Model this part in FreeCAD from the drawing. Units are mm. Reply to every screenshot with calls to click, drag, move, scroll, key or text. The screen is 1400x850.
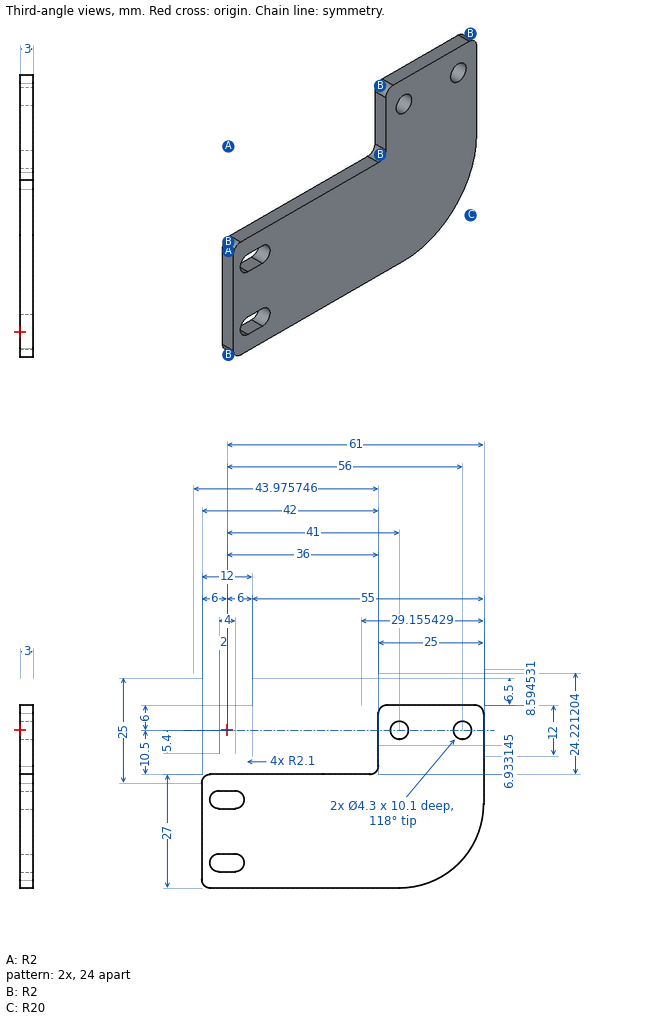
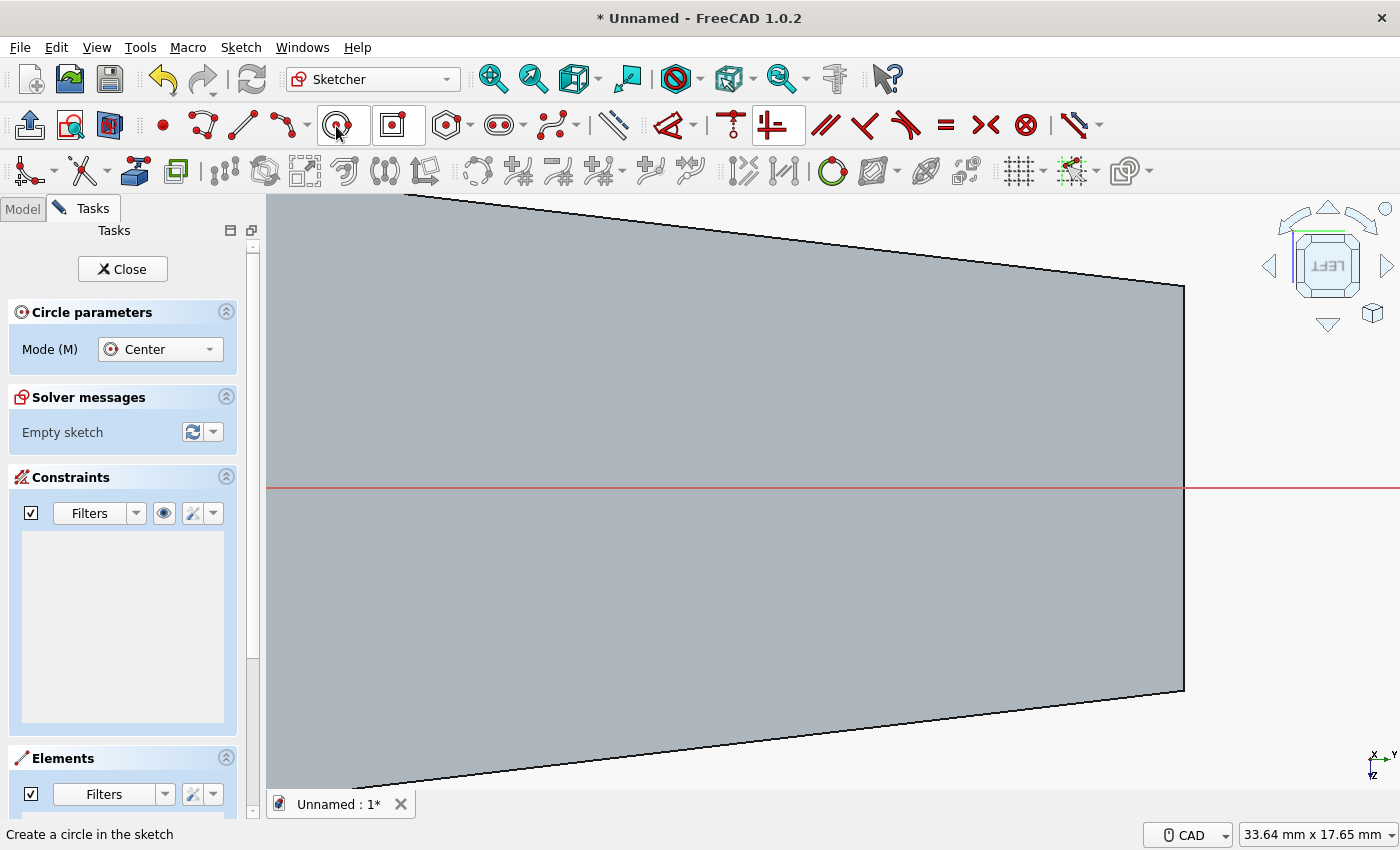
click(1016, 488)
move(1067, 437)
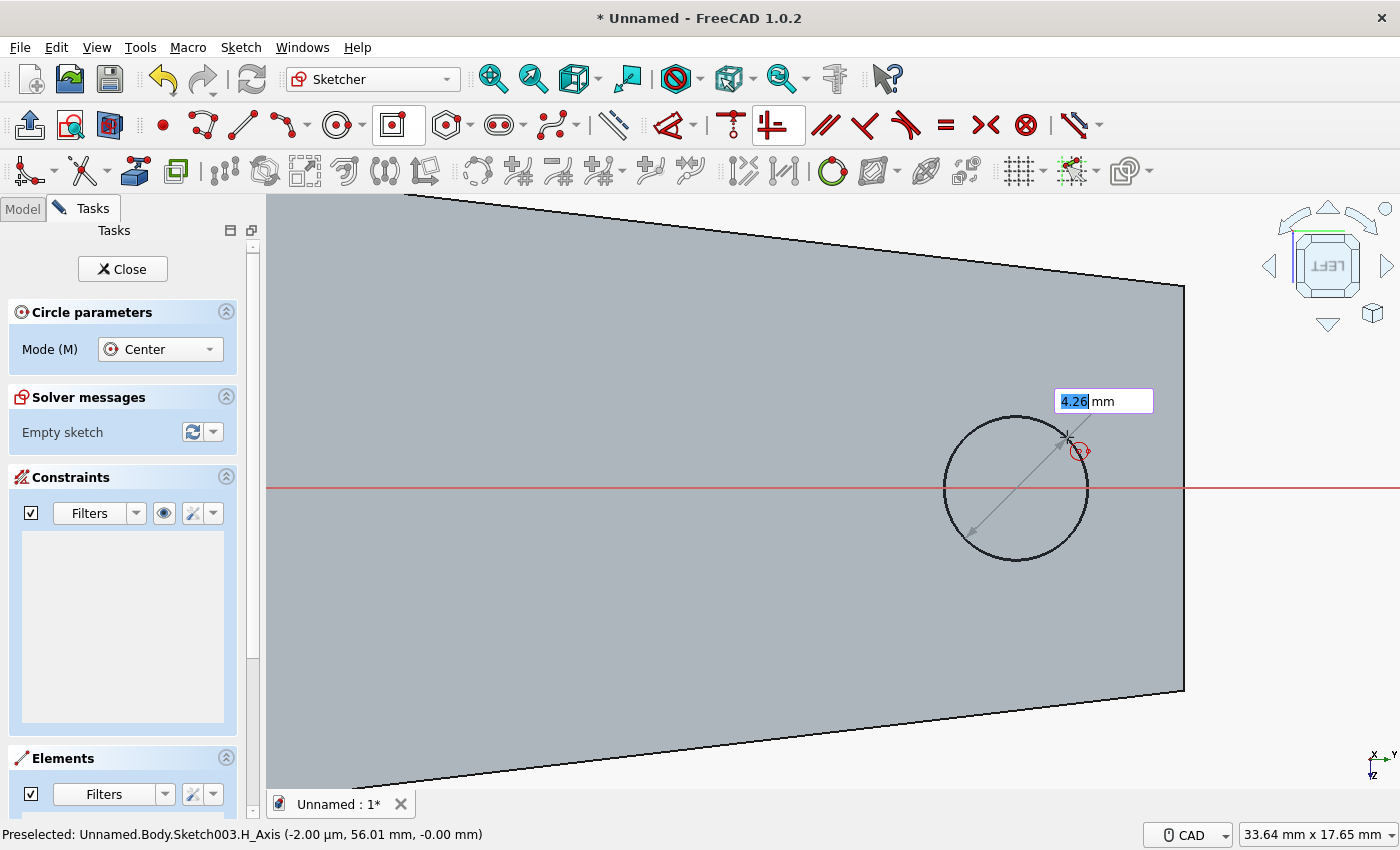
text(4.3)
key(Return)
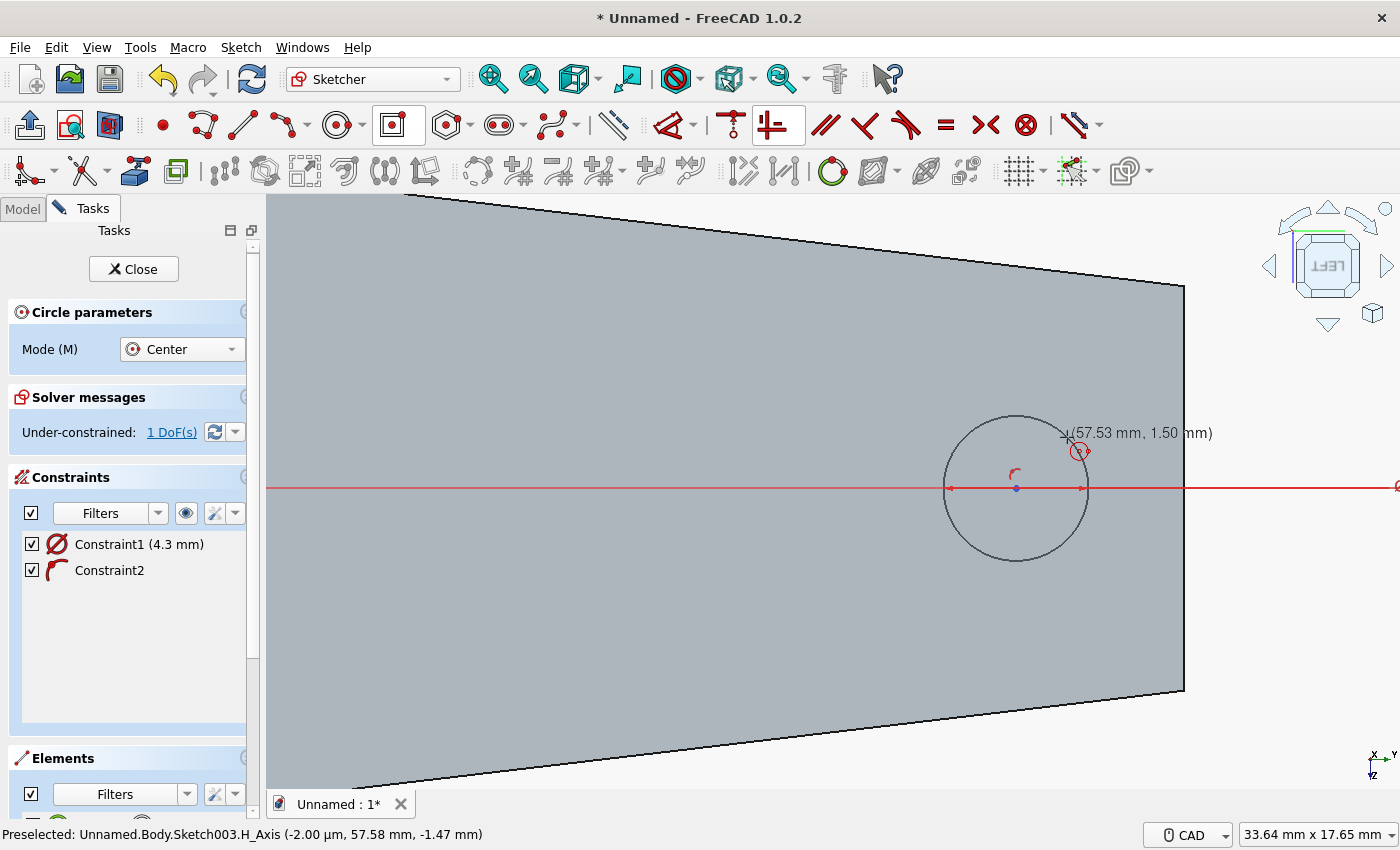
click(510, 488)
move(561, 437)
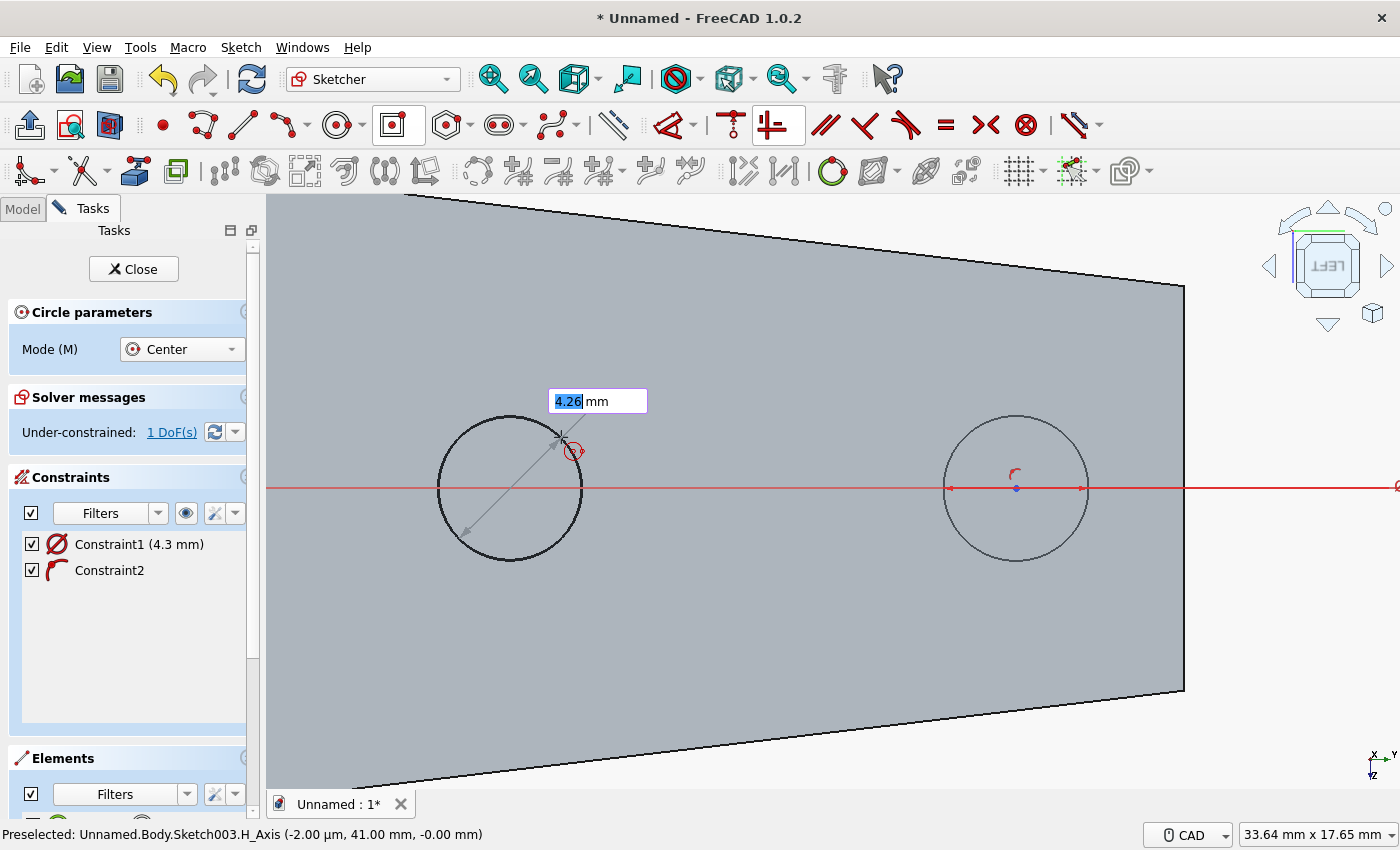
text(4.3)
key(Return)
key(Escape)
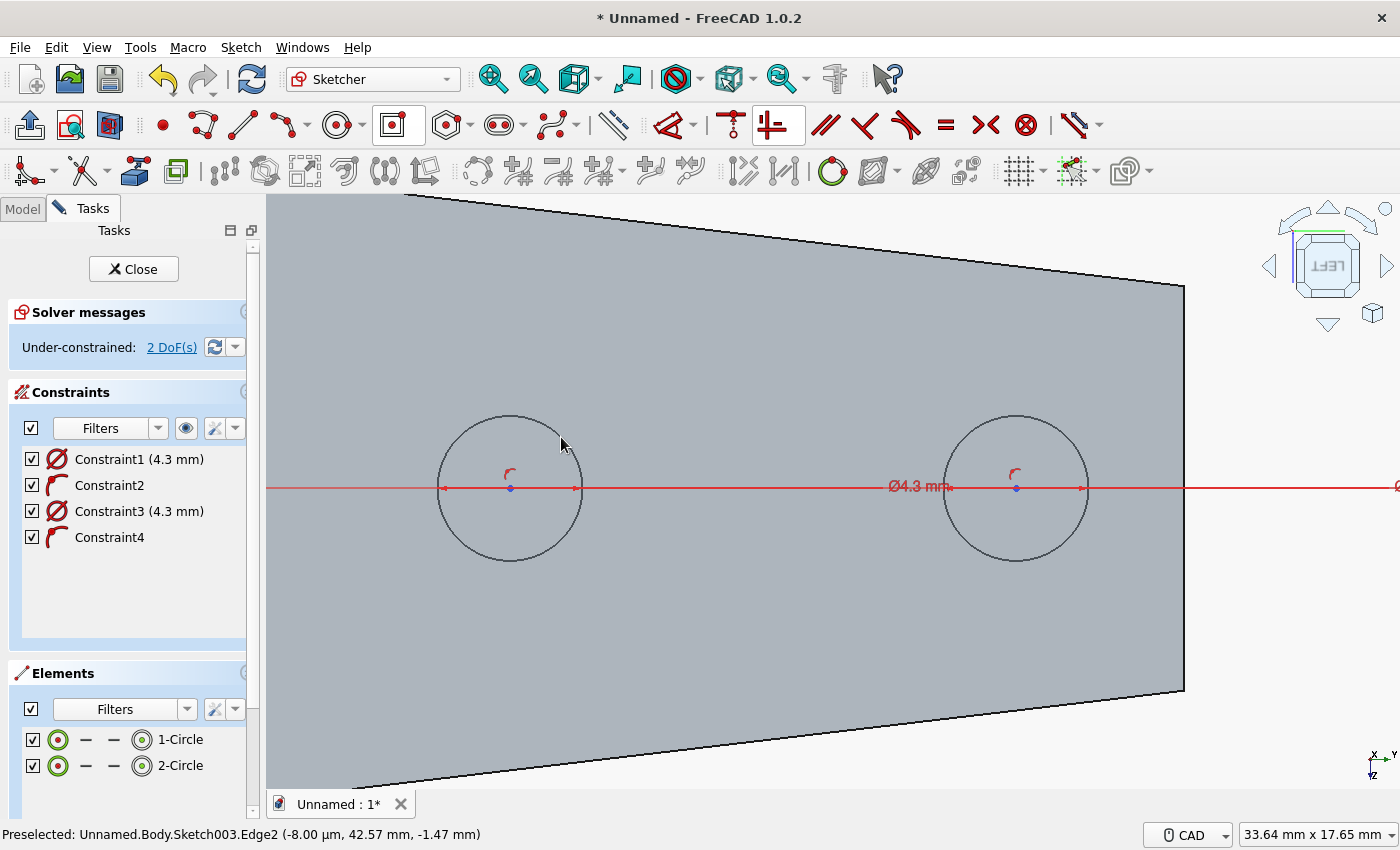
key(d)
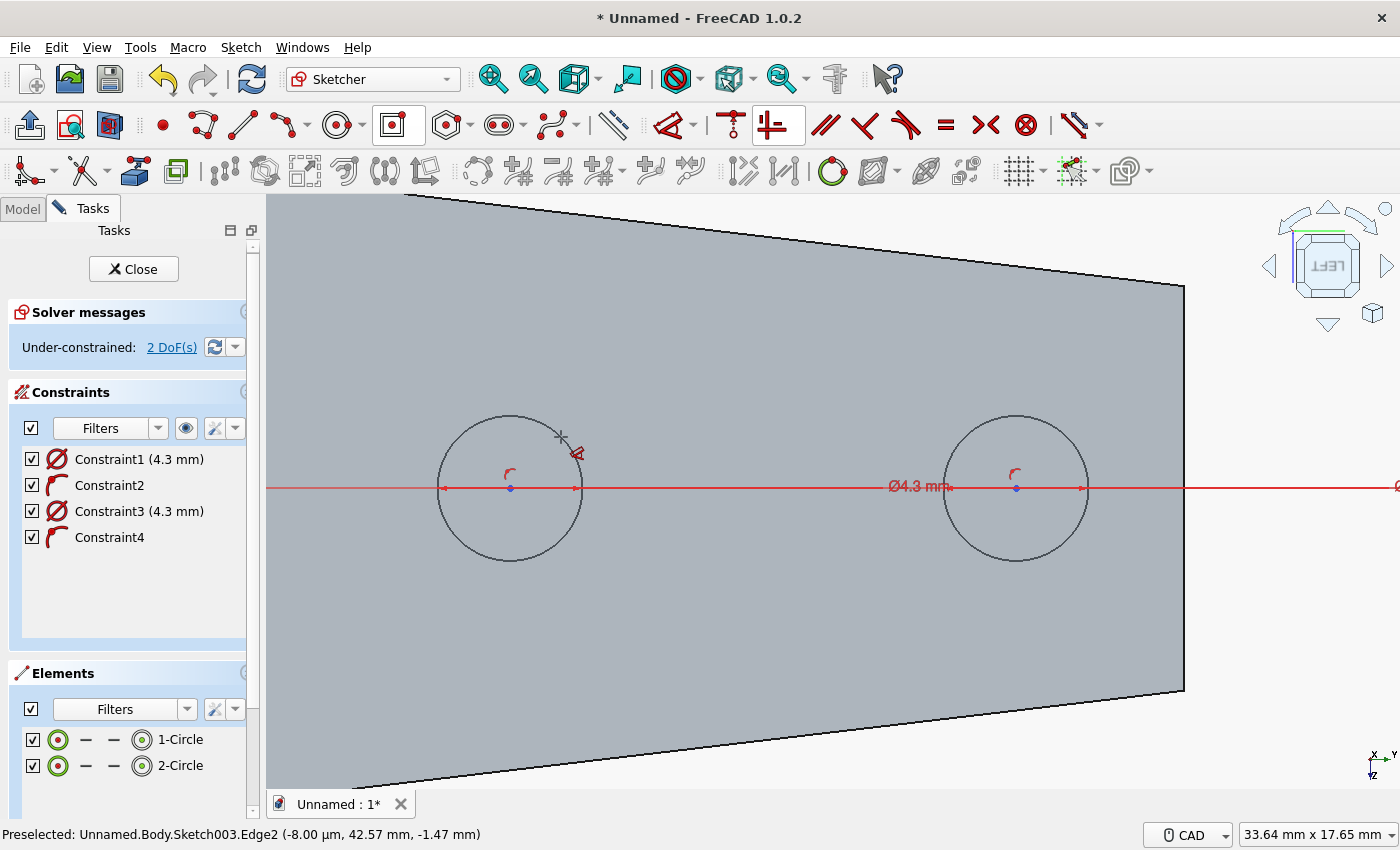
click(1016, 488)
click(655, 522)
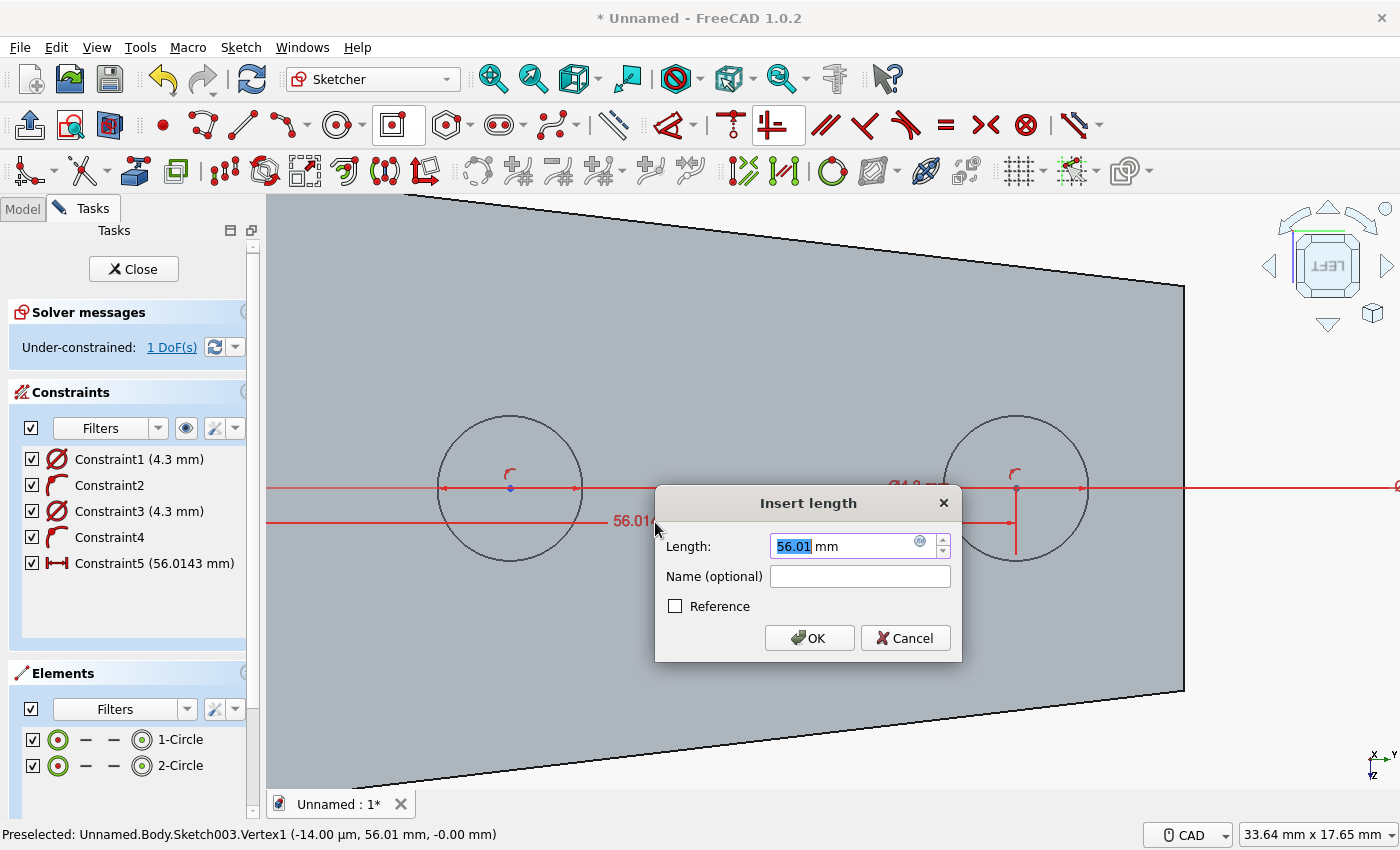
text(56)
key(Return)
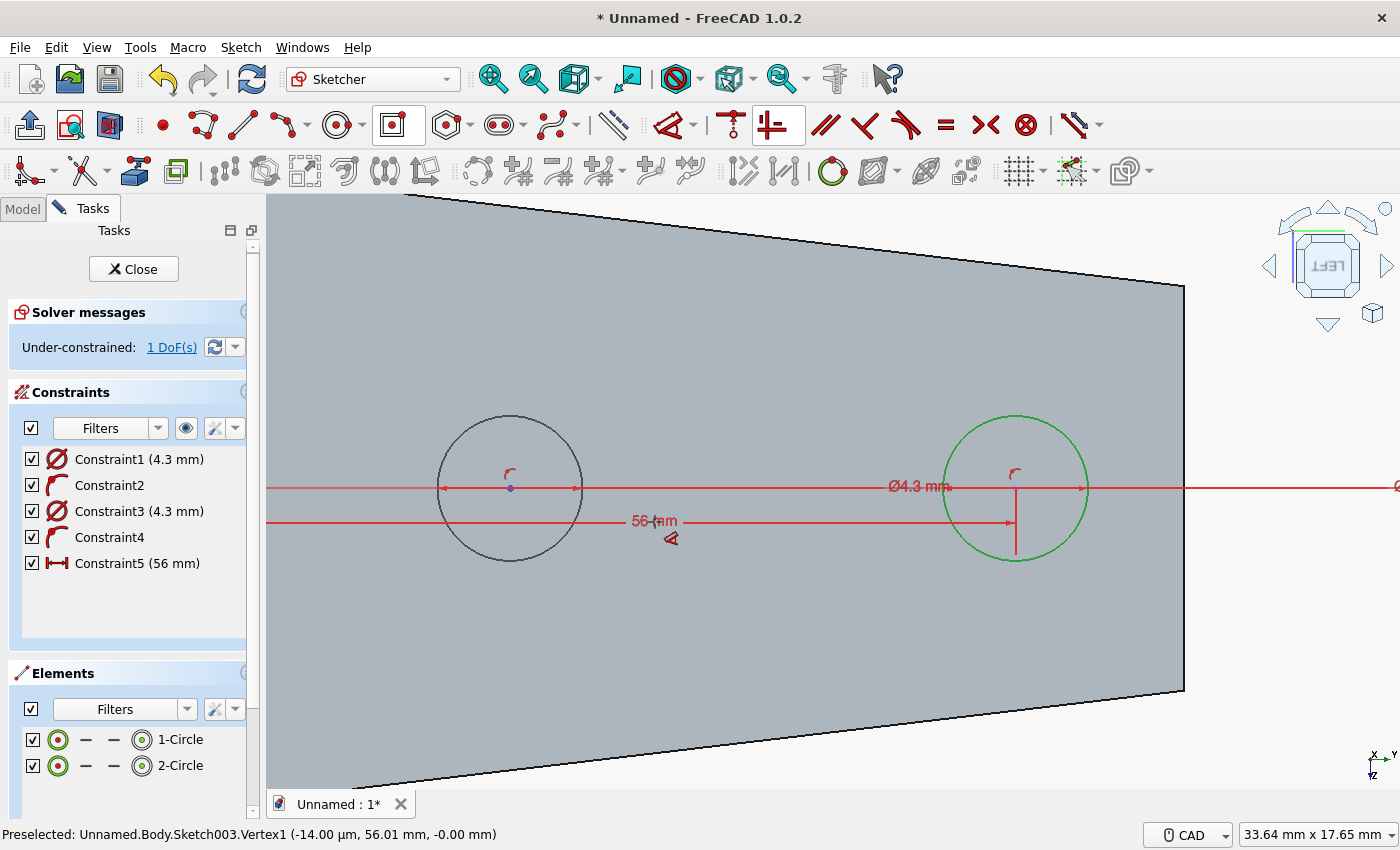
click(510, 488)
click(402, 522)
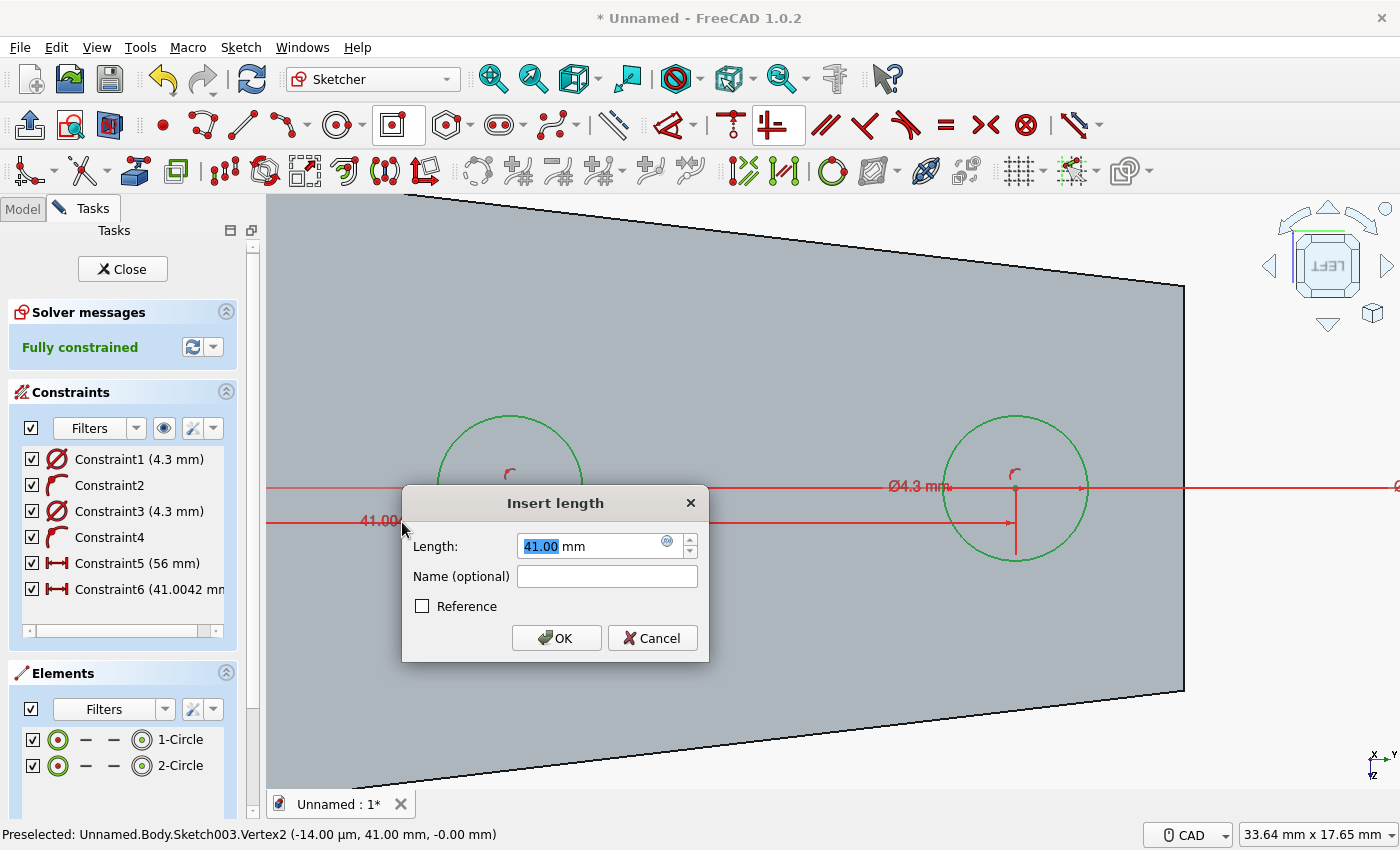
text(41)
key(Return)
key(Escape)